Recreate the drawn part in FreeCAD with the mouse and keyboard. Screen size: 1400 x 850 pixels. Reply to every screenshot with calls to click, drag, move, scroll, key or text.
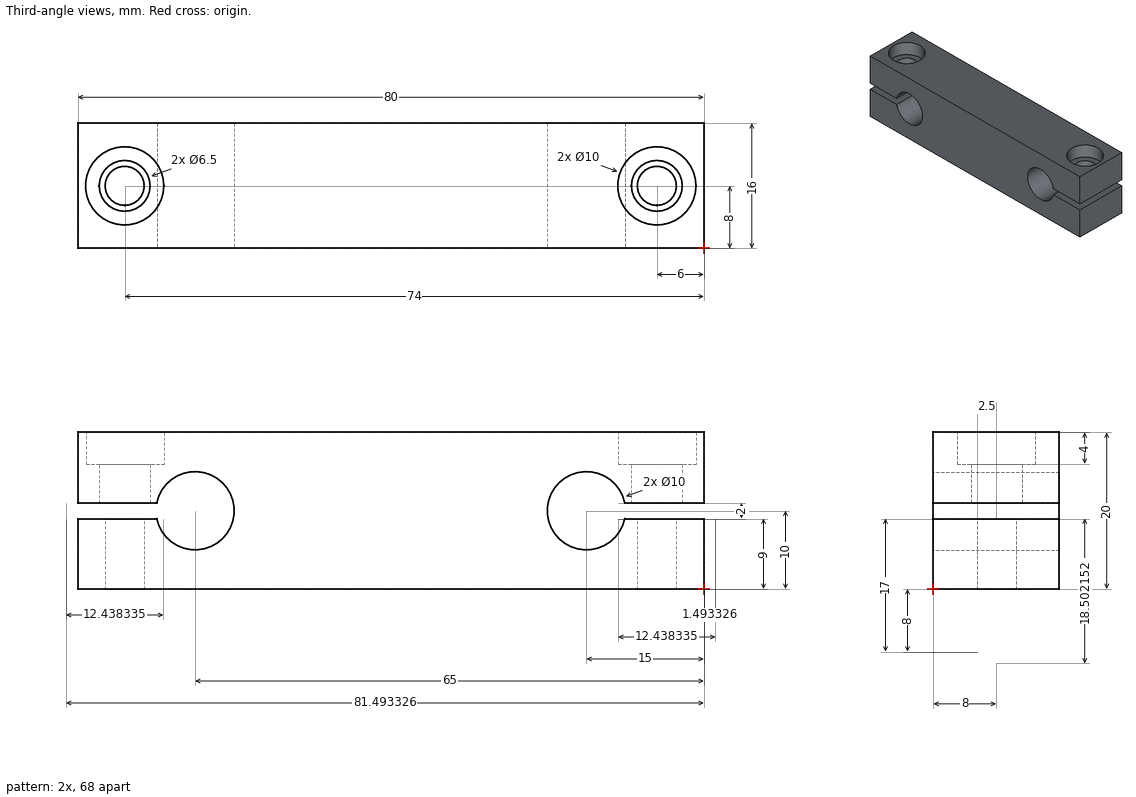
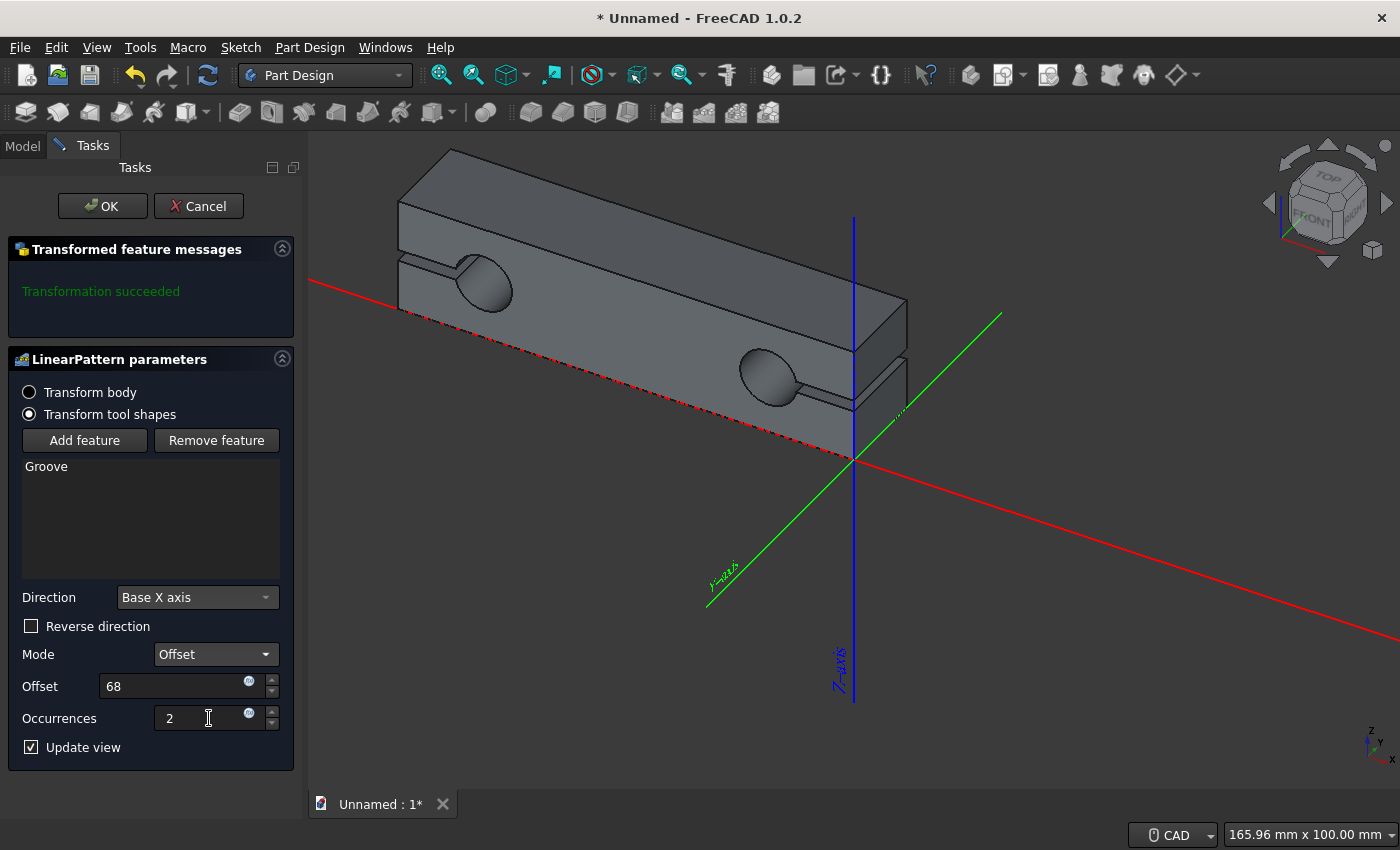
click(30, 626)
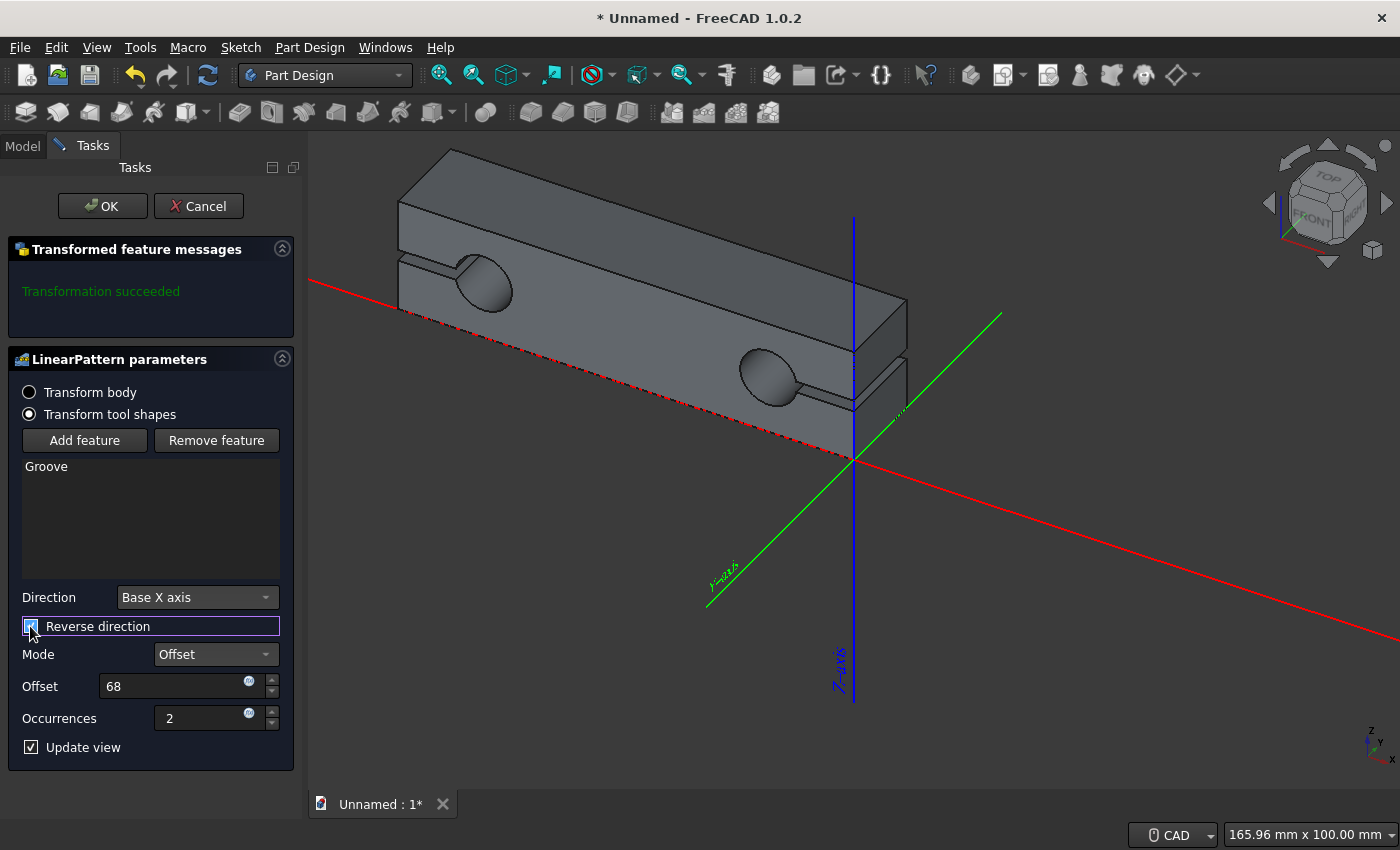
click(103, 206)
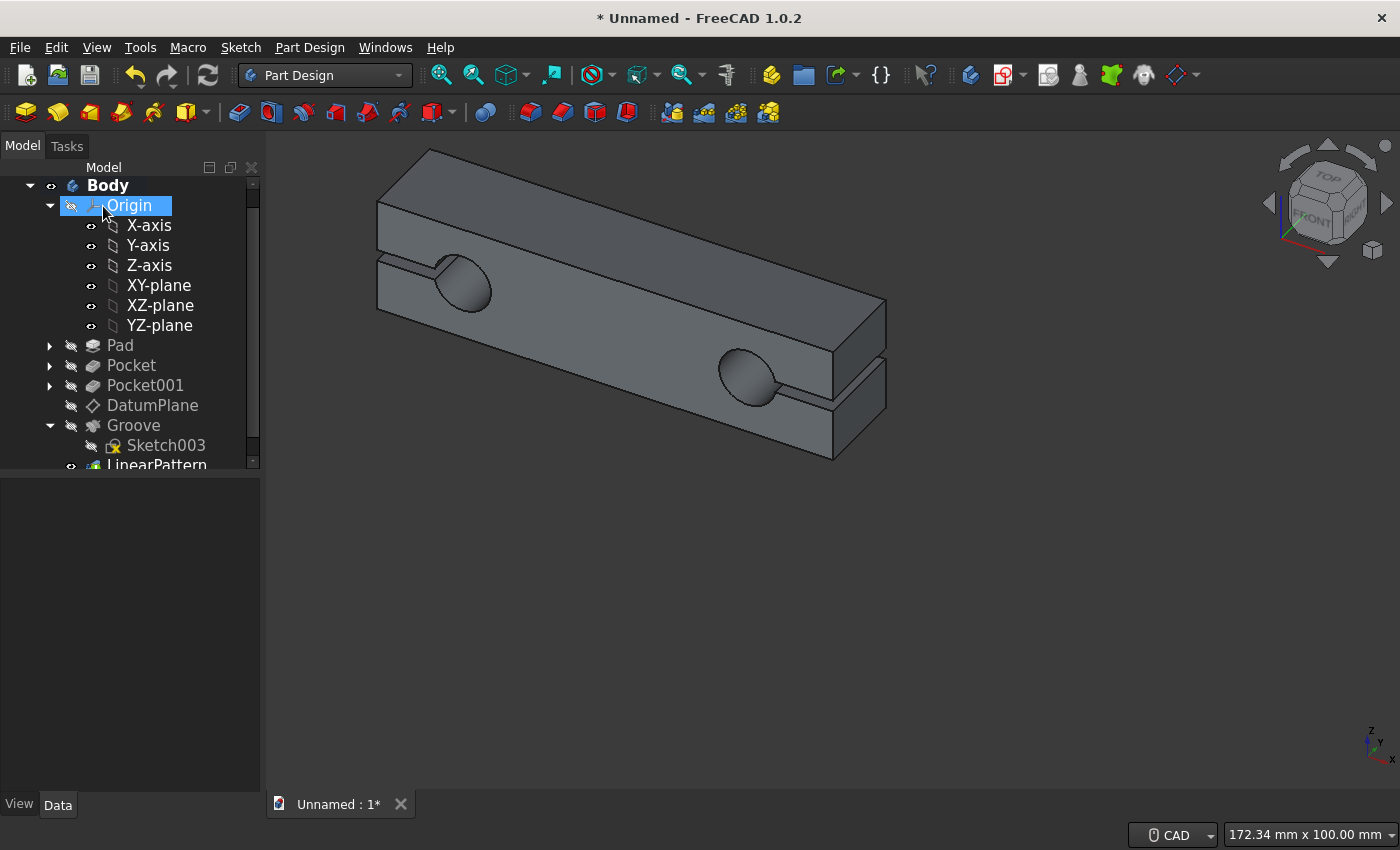
key(5)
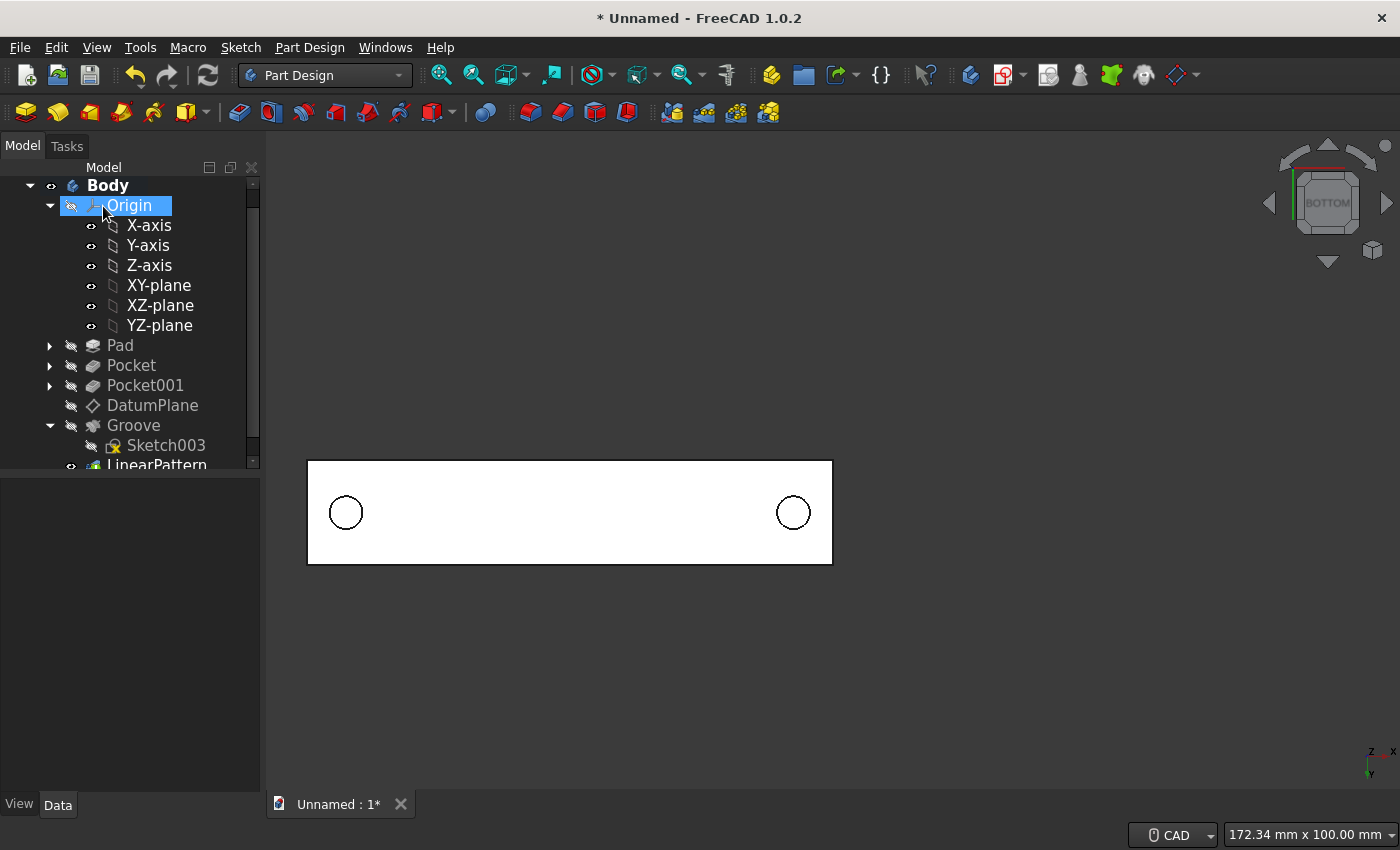
click(800, 512)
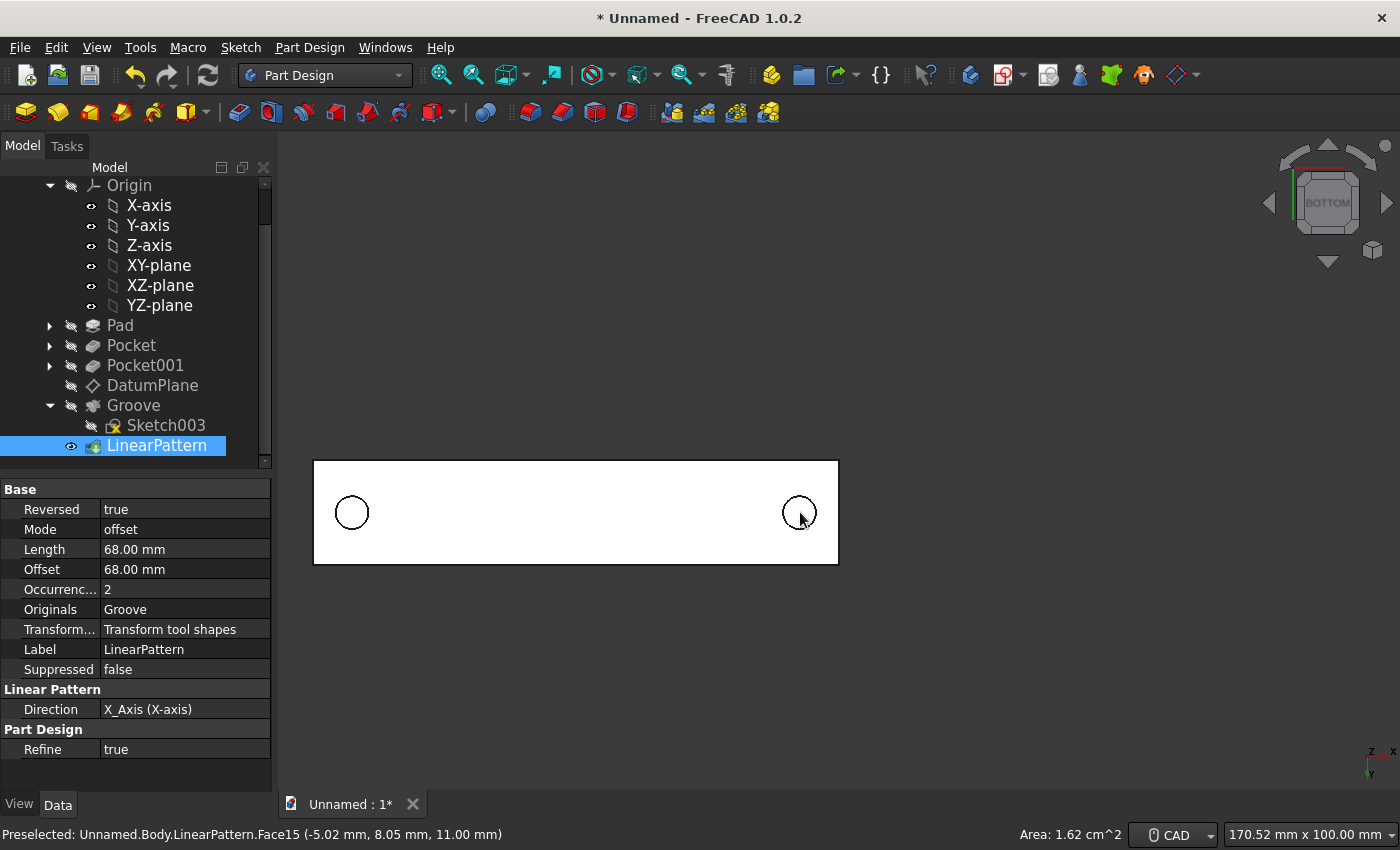
click(1004, 76)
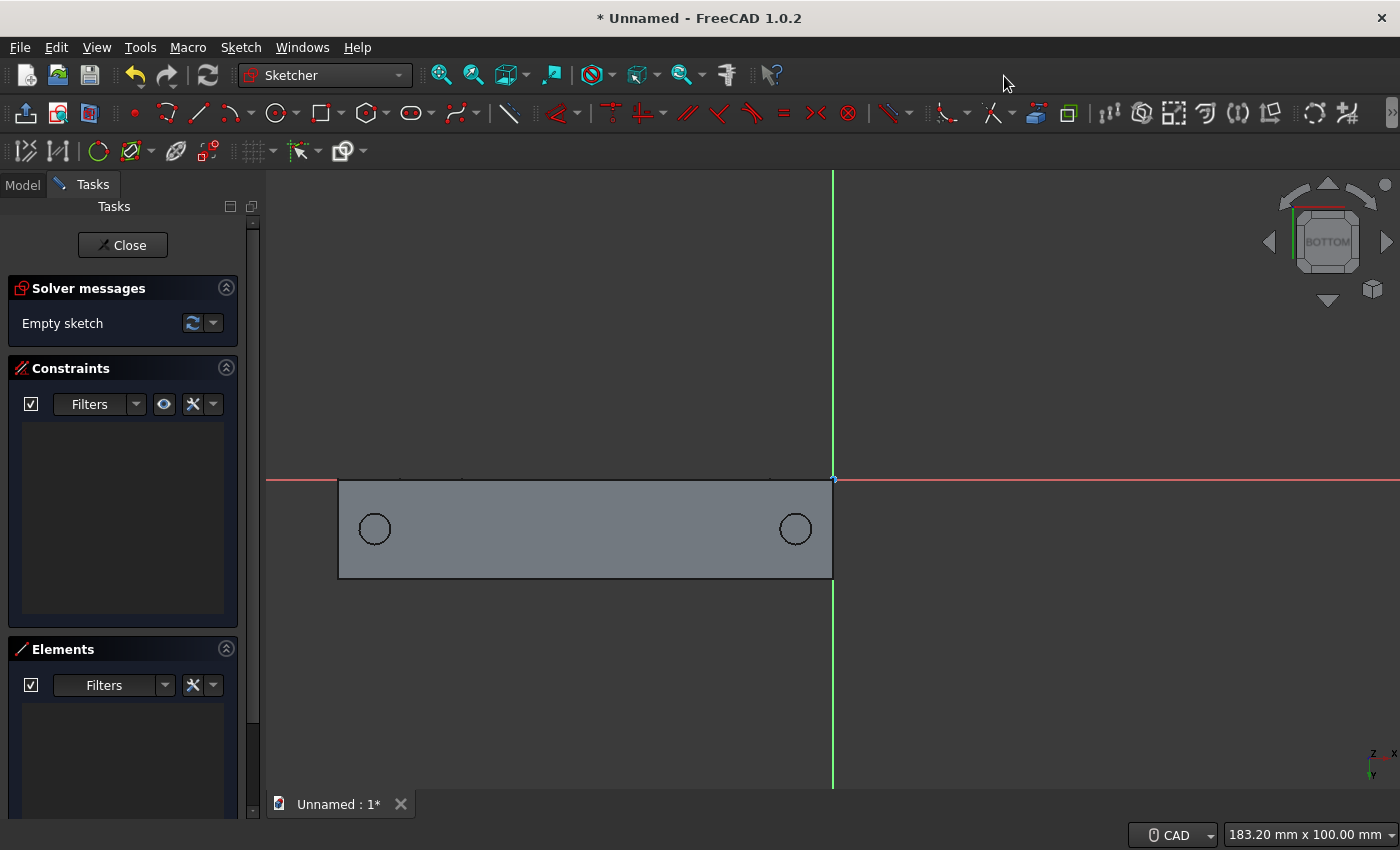
click(90, 114)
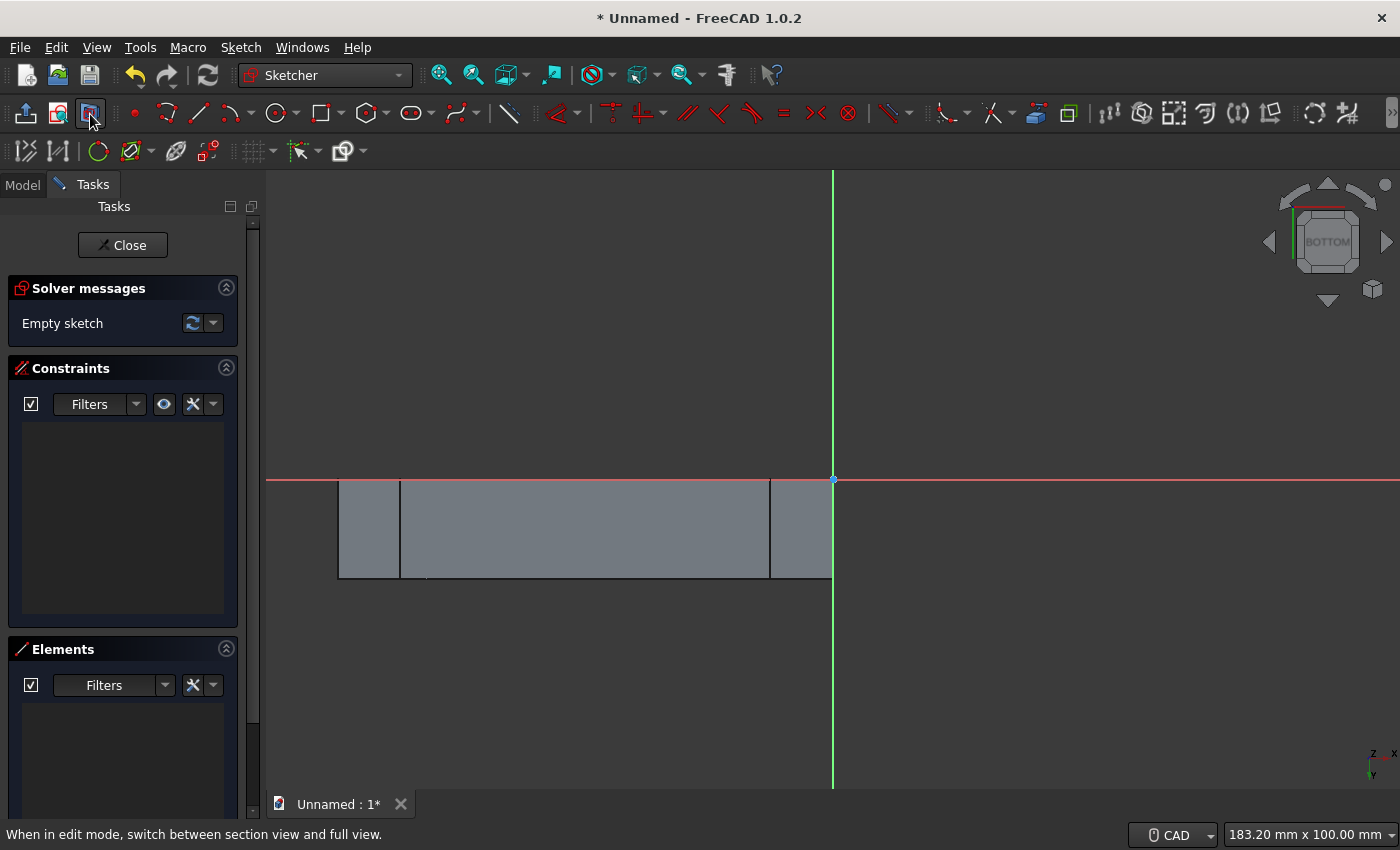
scroll(294, 585, up, 2)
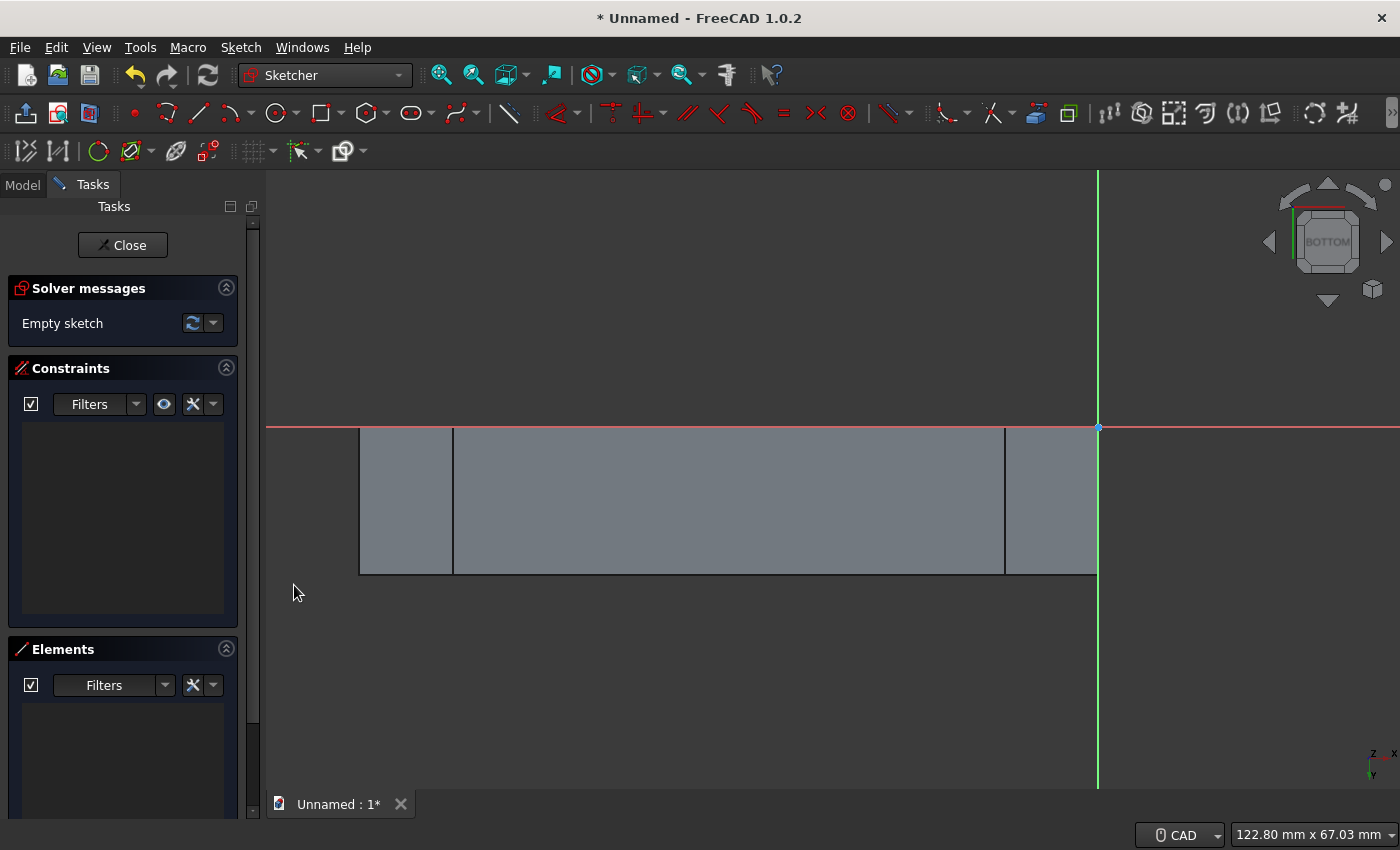
click(276, 114)